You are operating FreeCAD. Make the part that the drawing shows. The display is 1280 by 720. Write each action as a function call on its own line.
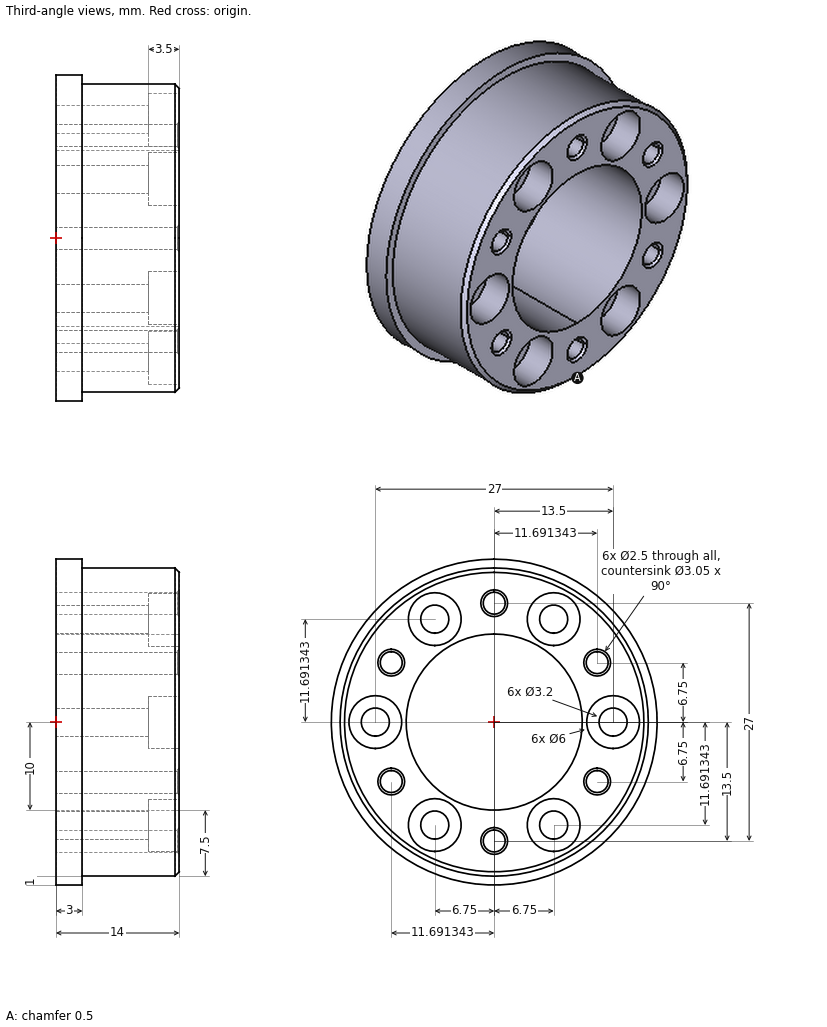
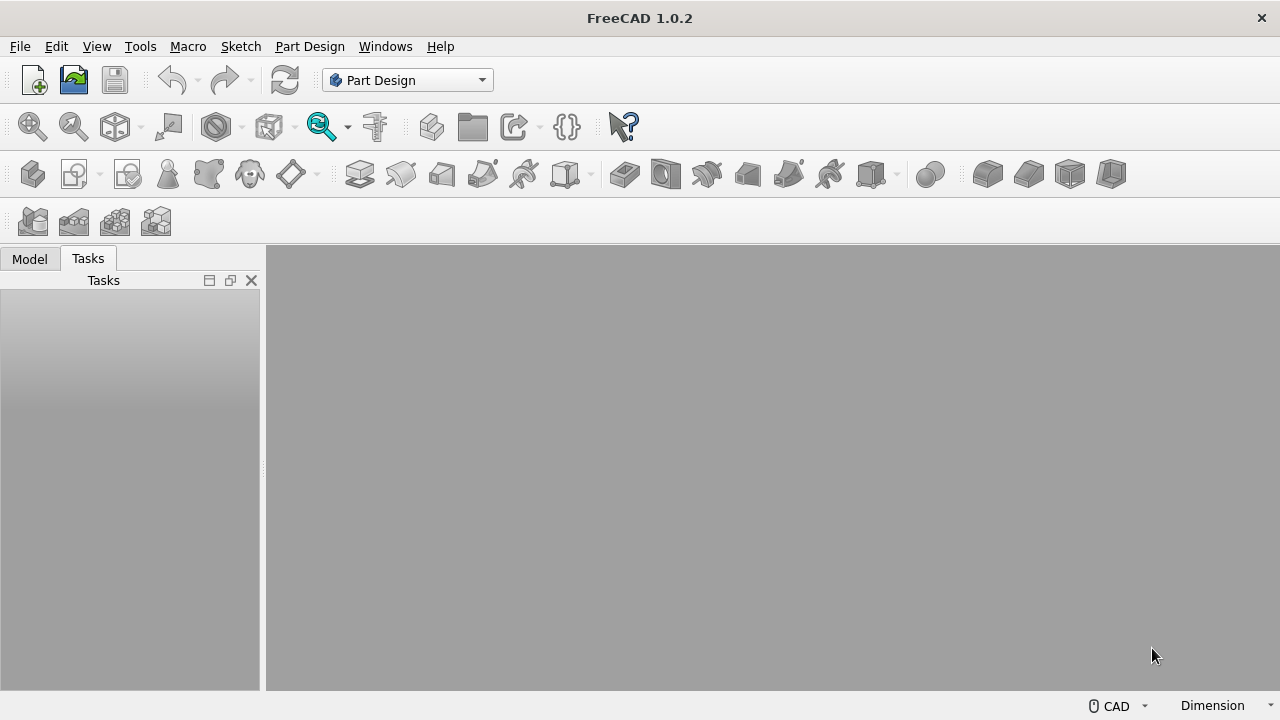
click(33, 80)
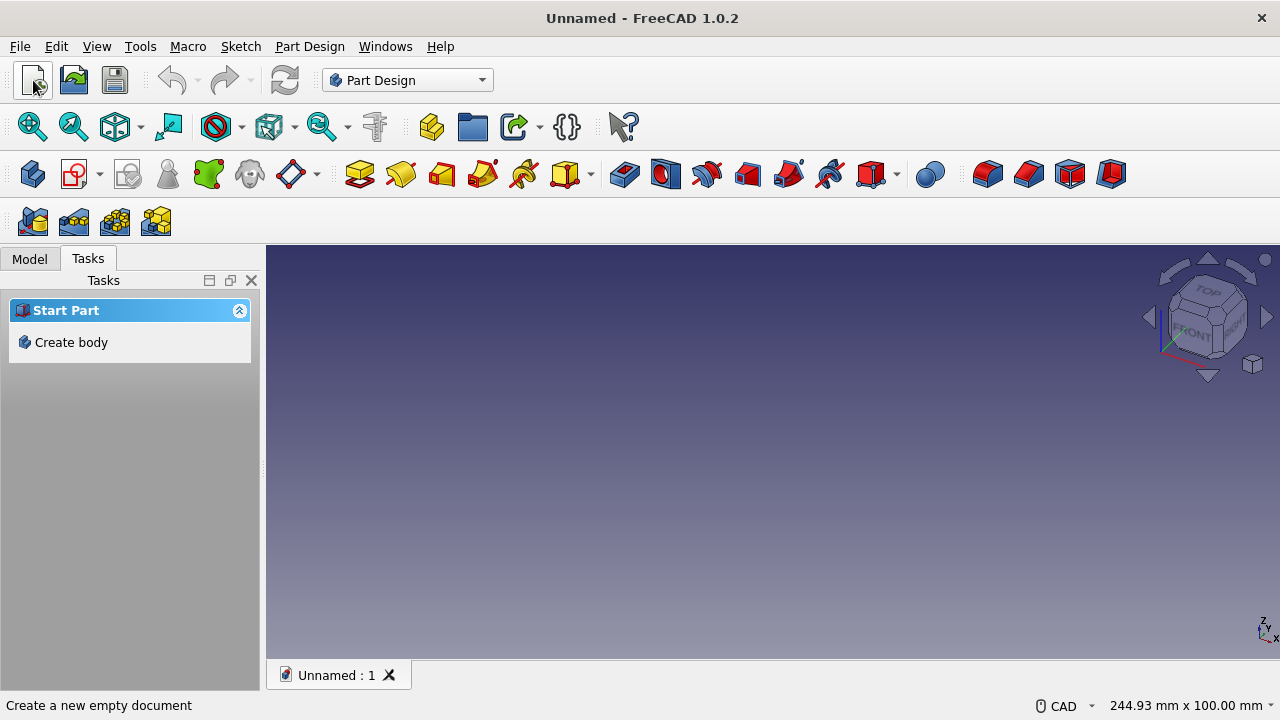
click(74, 174)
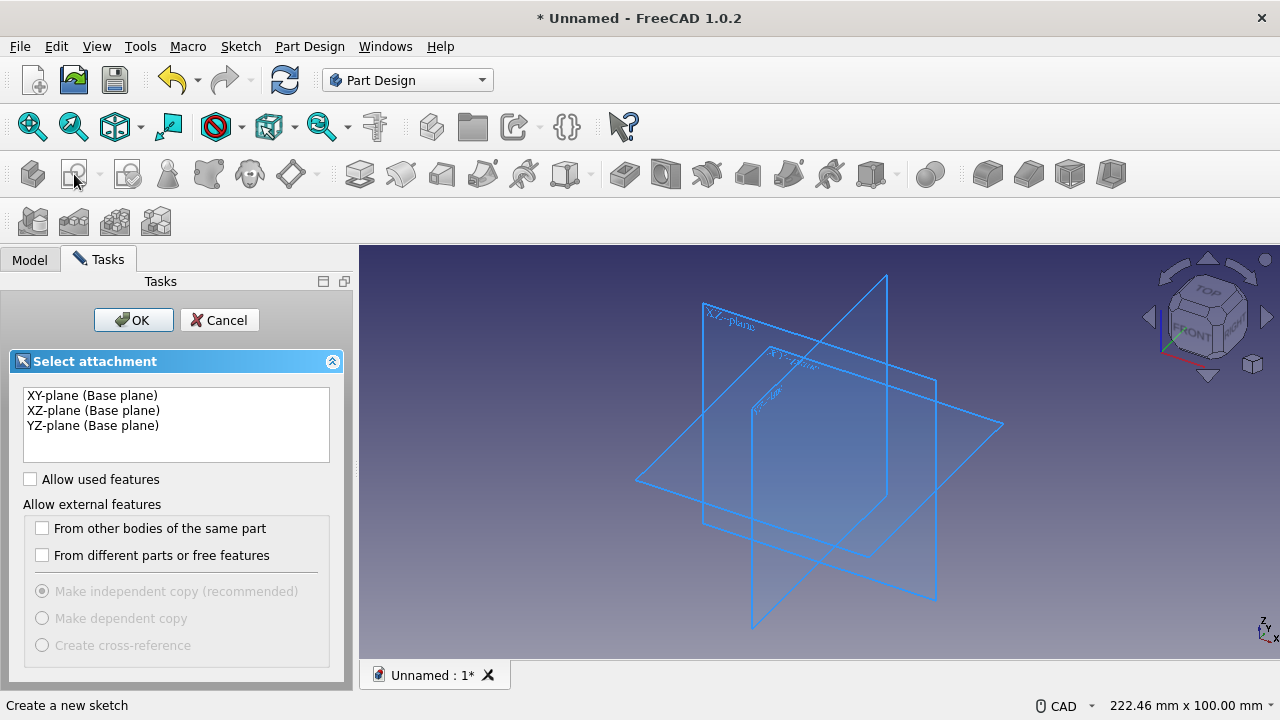
click(84, 410)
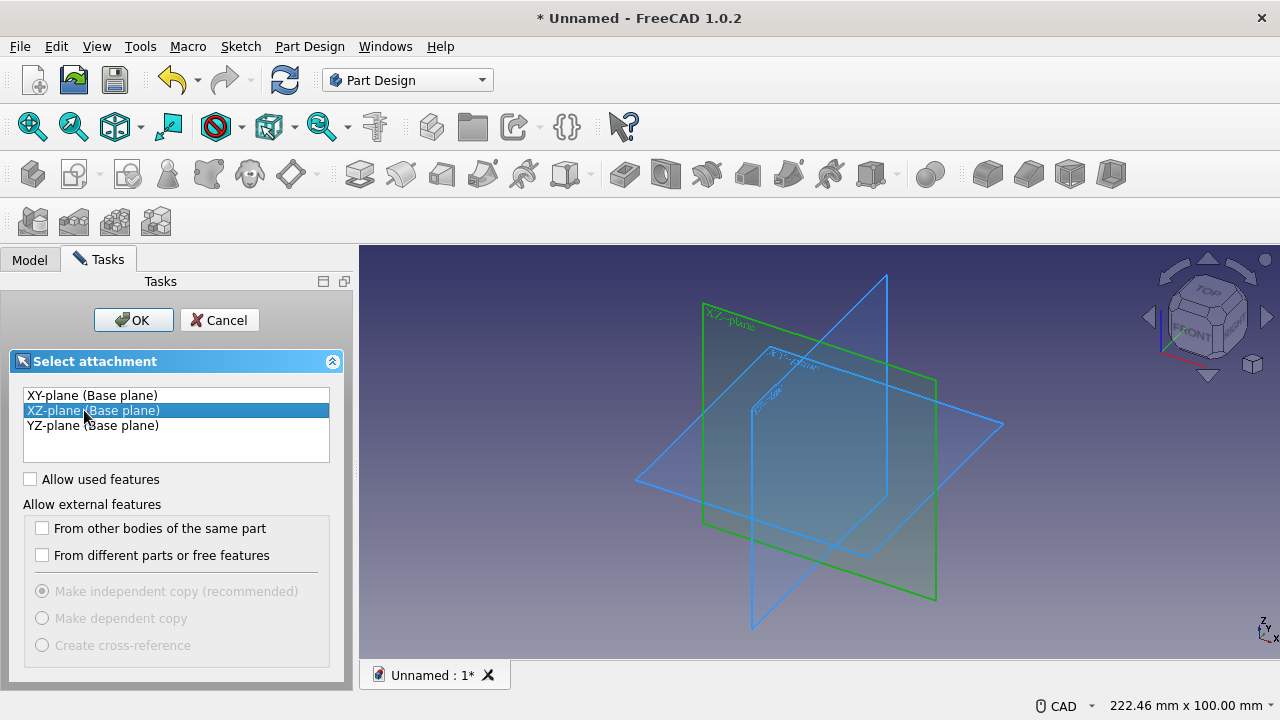
click(134, 320)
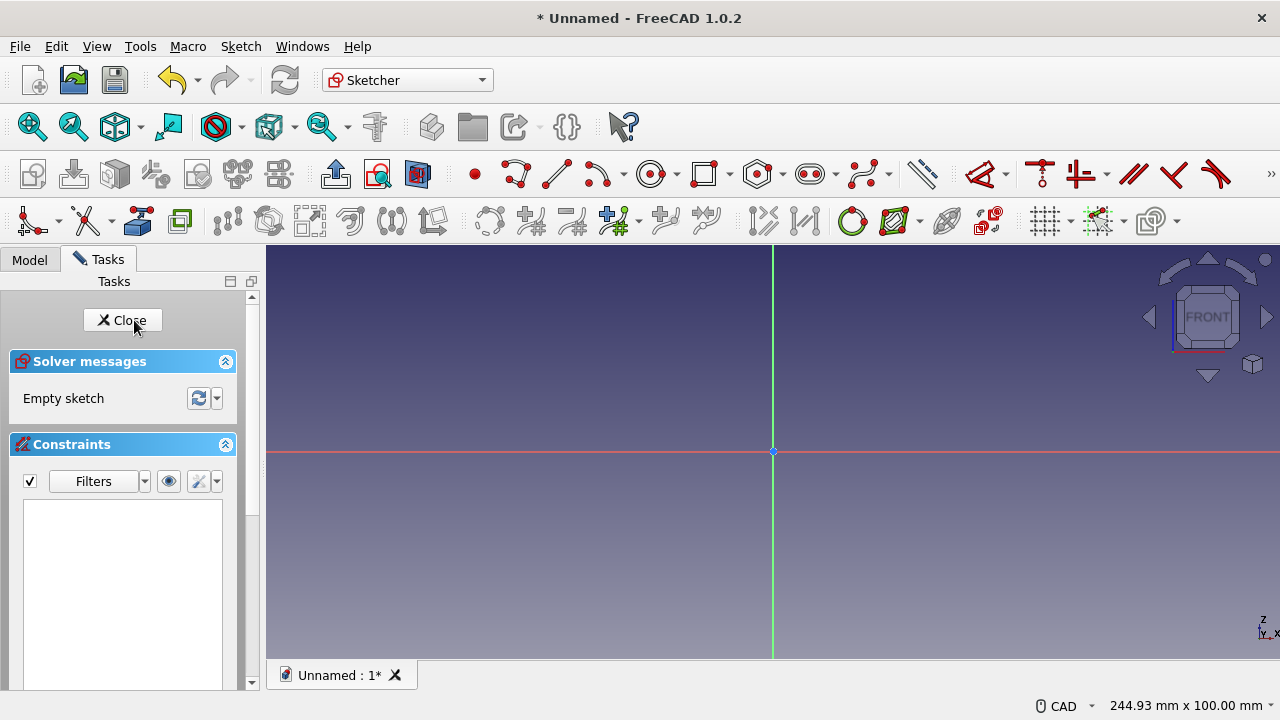
scroll(844, 507, up, 6)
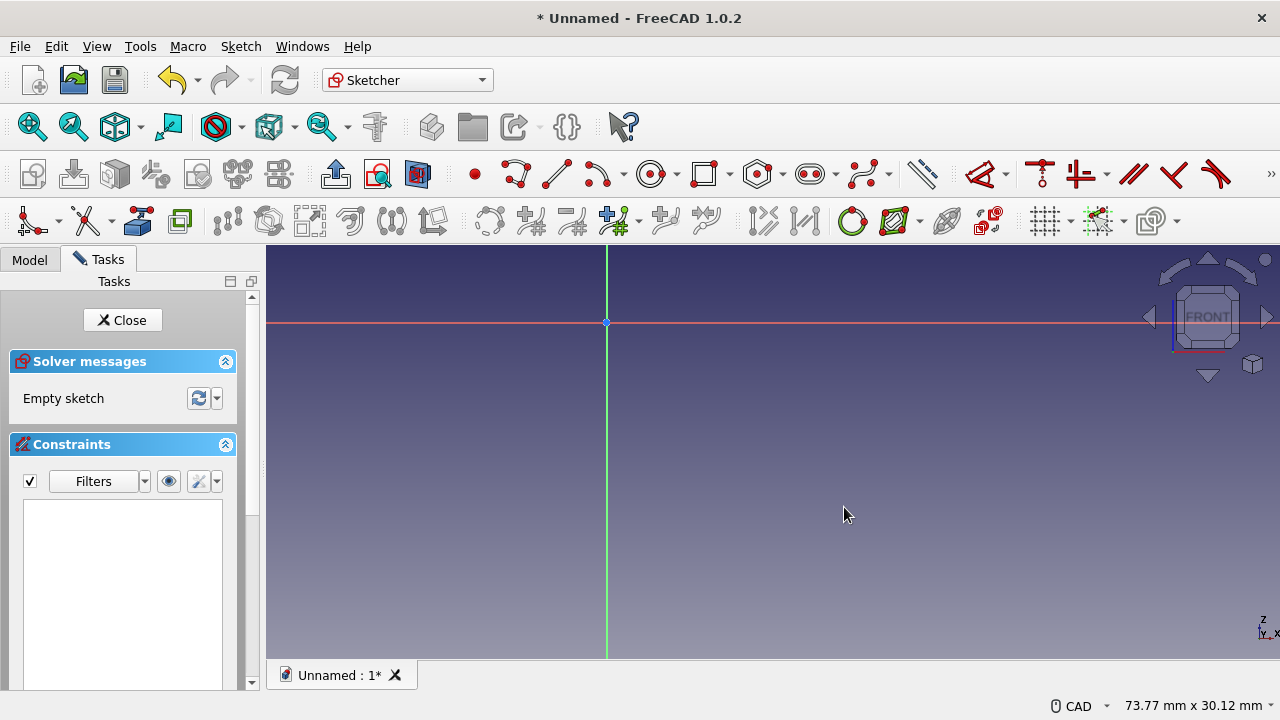
click(516, 174)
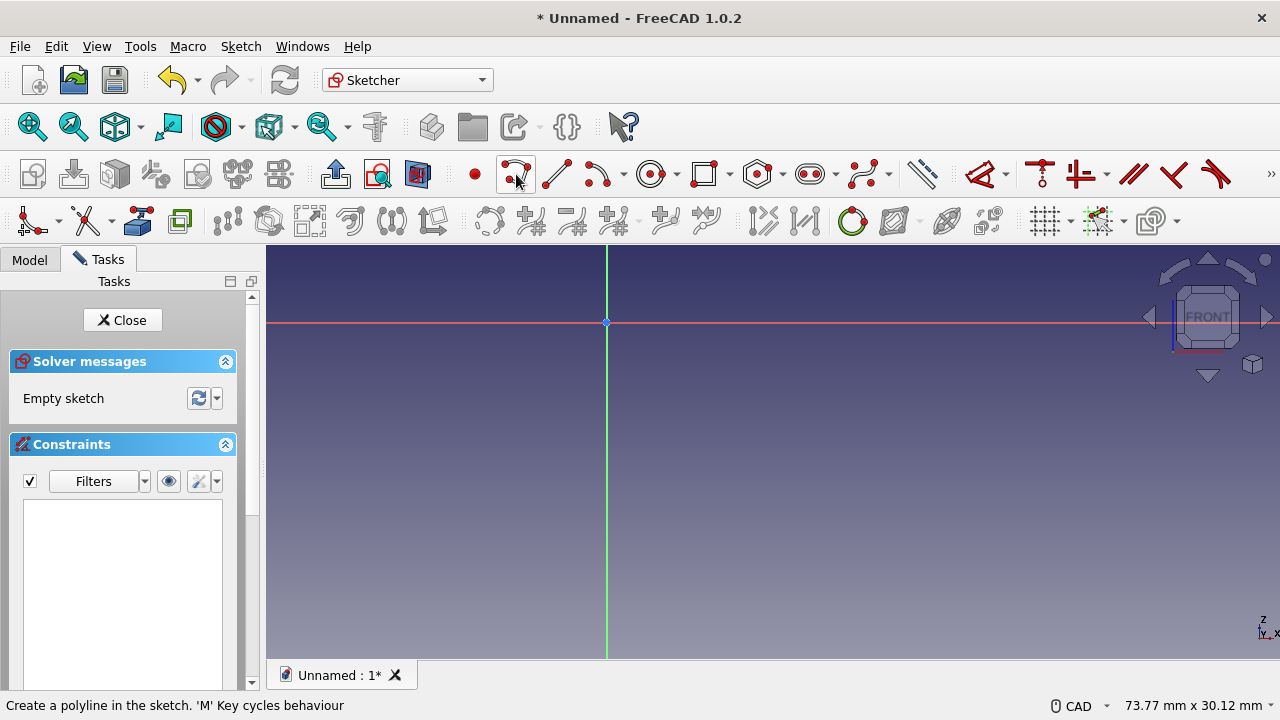
click(607, 460)
click(799, 460)
click(799, 563)
click(648, 563)
click(648, 577)
click(616, 577)
click(607, 461)
key(Escape)
key(Escape)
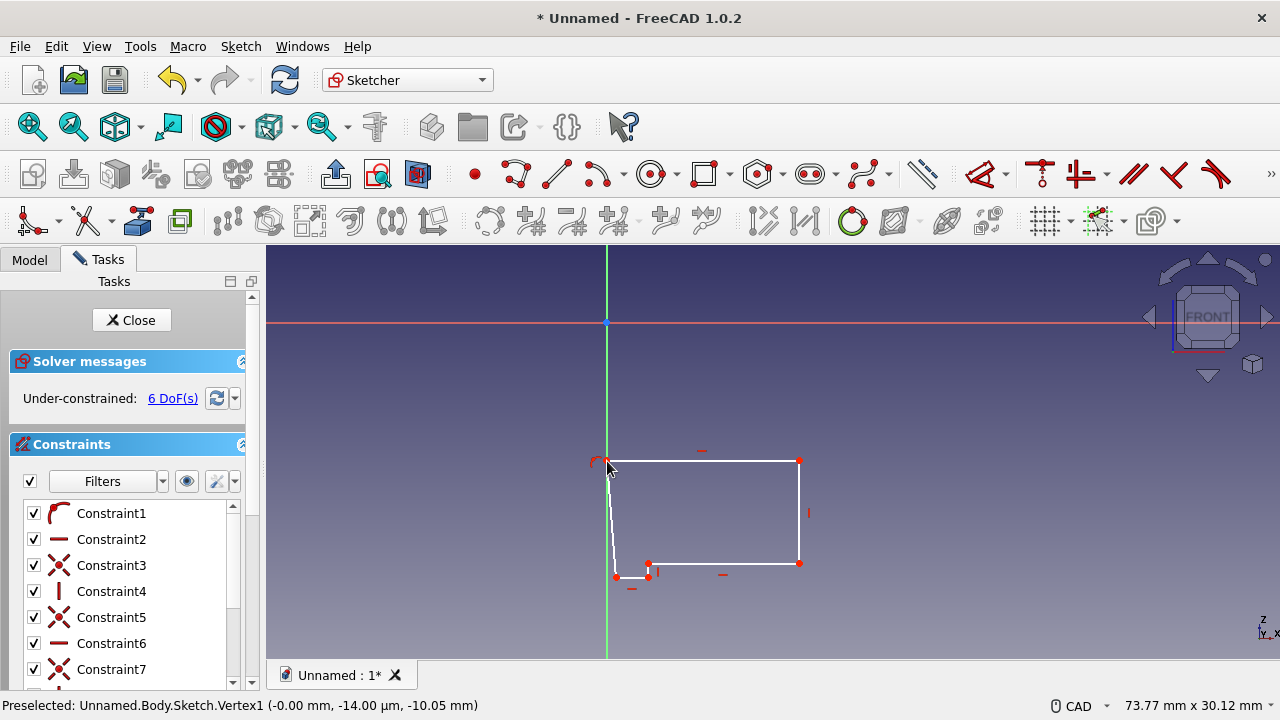
click(610, 496)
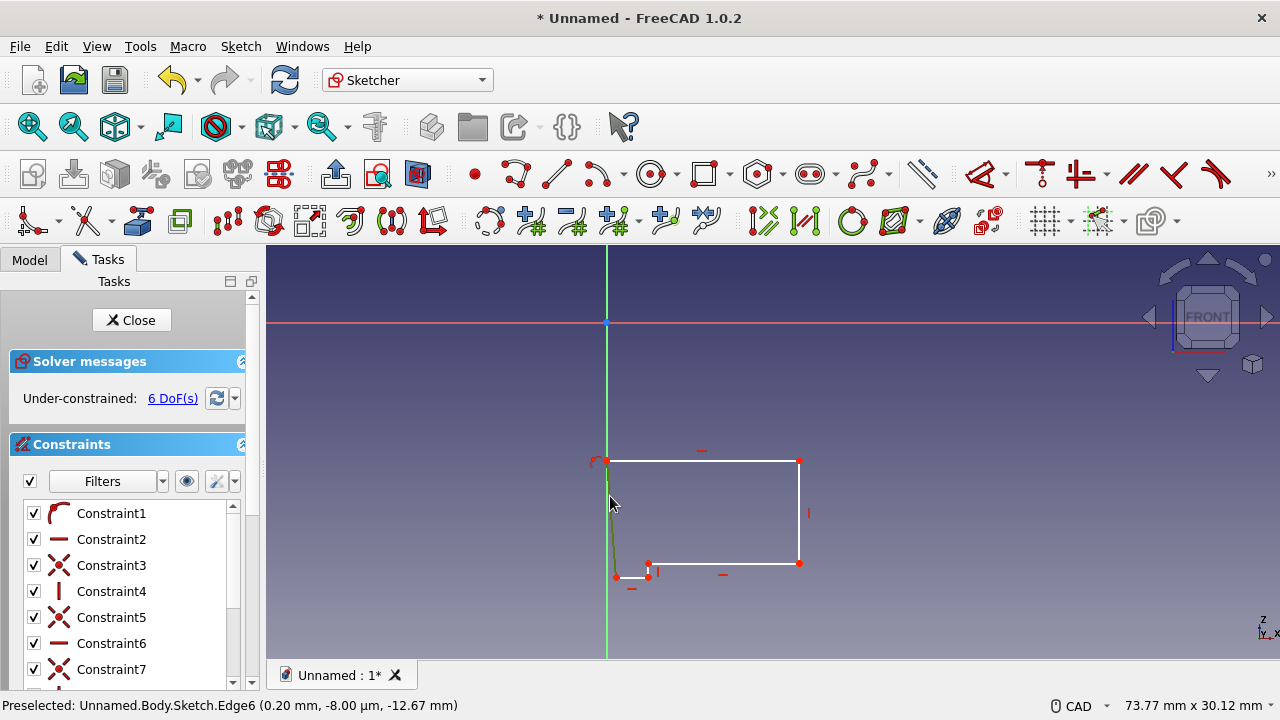
click(1106, 174)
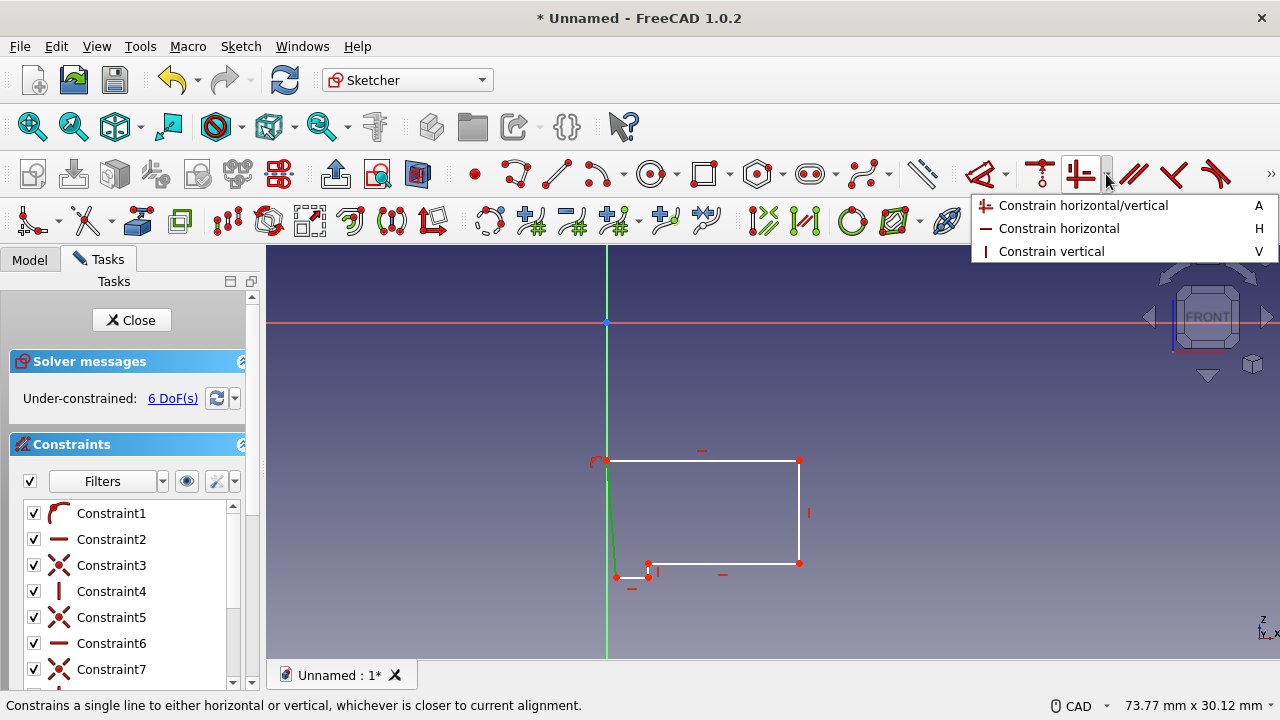
click(1125, 252)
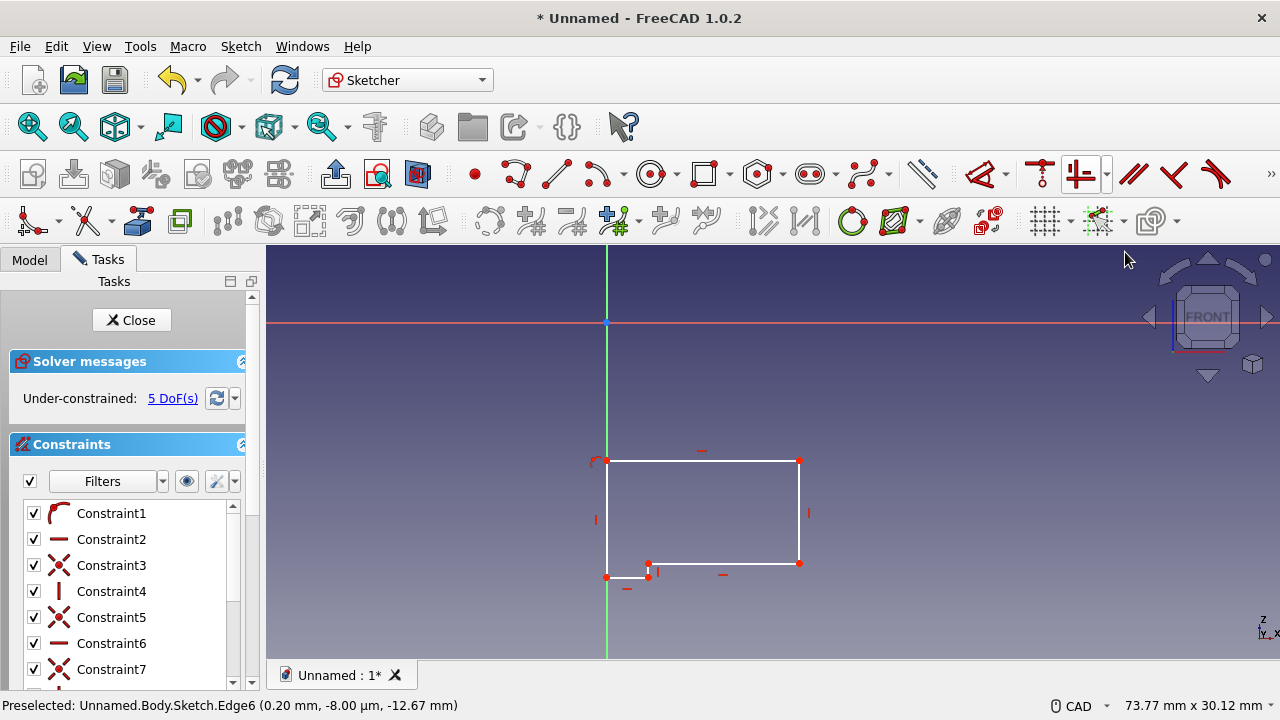
click(980, 174)